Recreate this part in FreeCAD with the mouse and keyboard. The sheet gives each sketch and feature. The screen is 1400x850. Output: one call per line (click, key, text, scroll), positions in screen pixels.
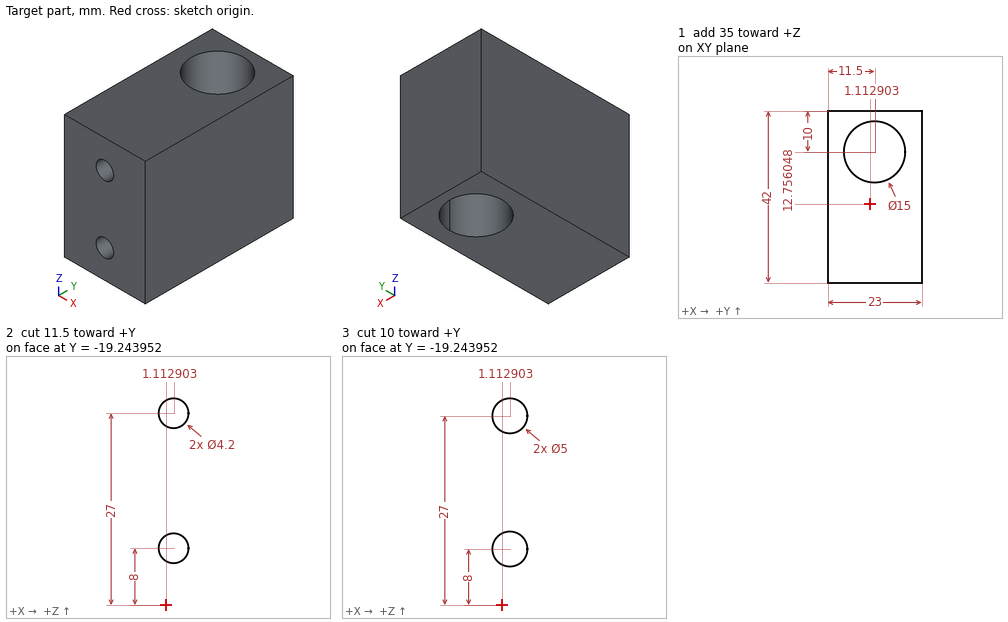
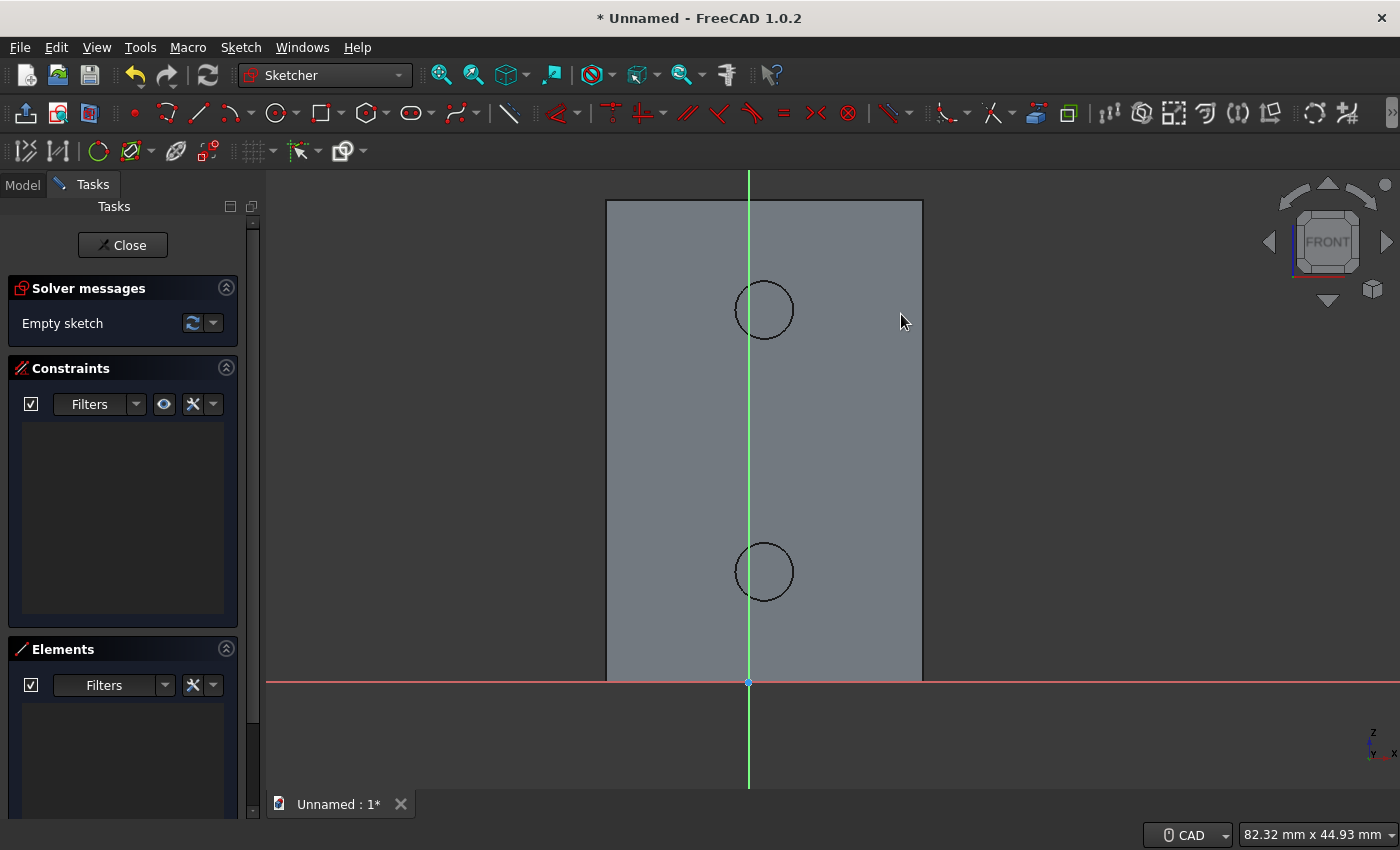
click(276, 114)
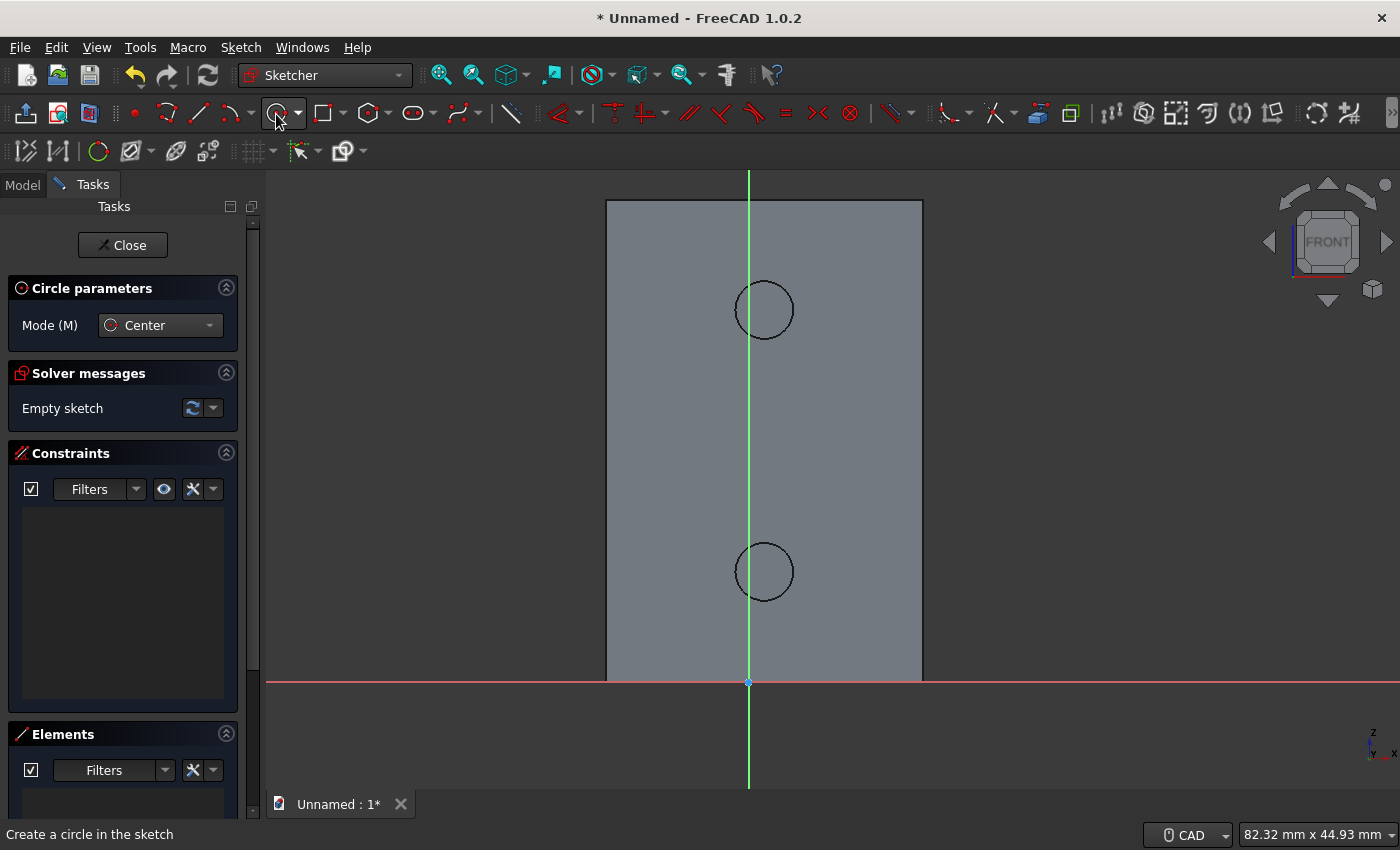
click(764, 310)
click(789, 286)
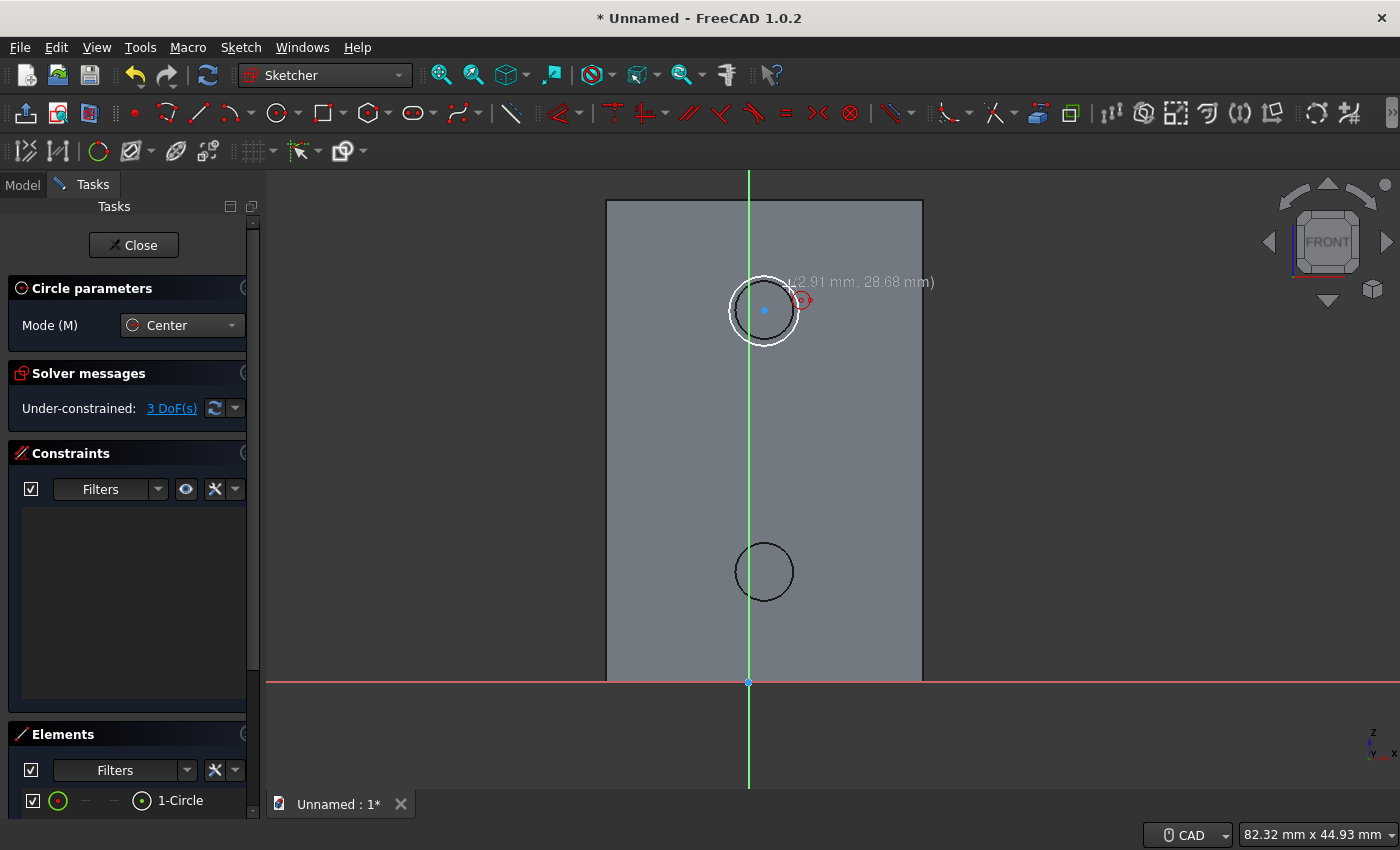
click(764, 572)
click(789, 547)
key(Escape)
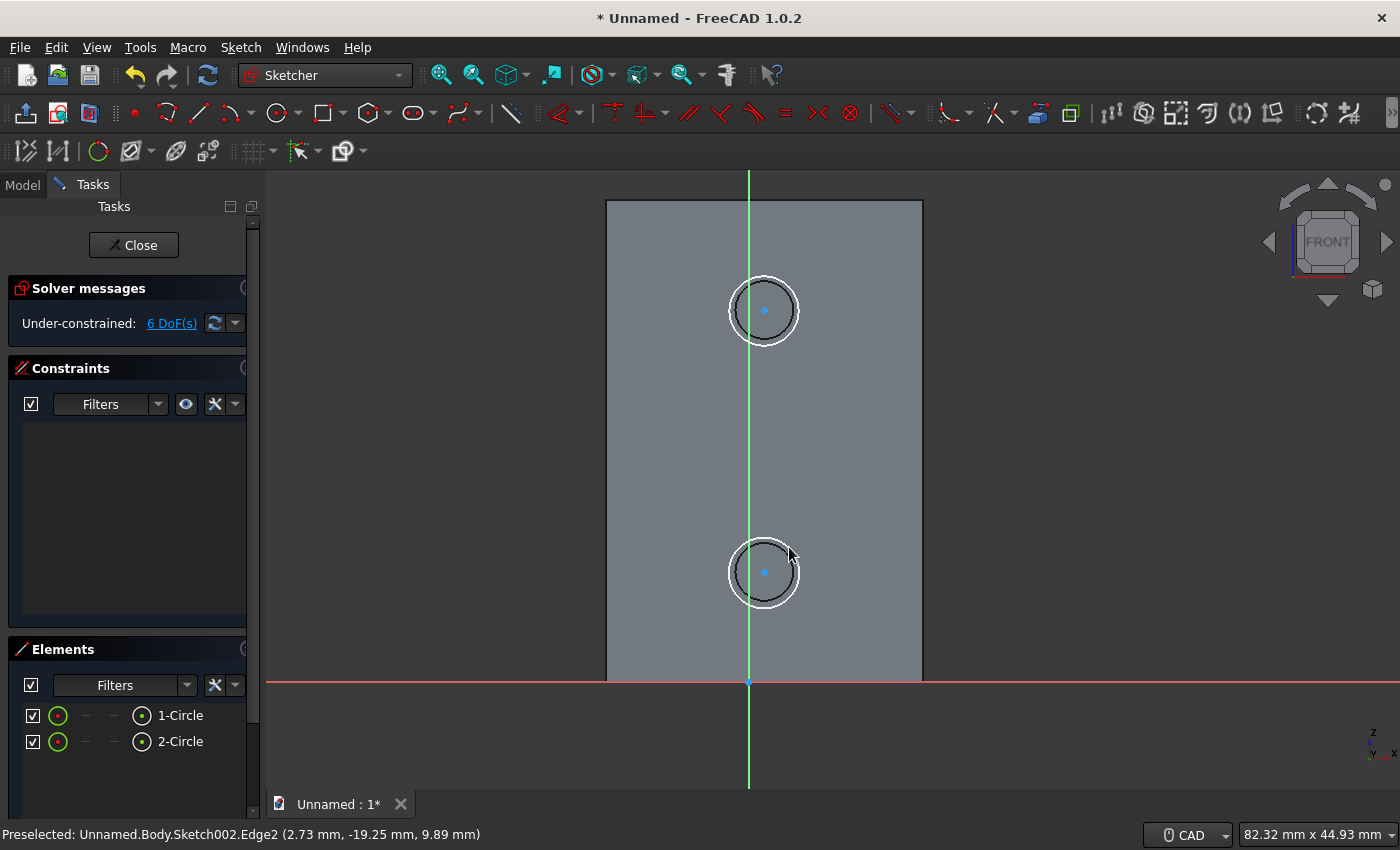
click(788, 286)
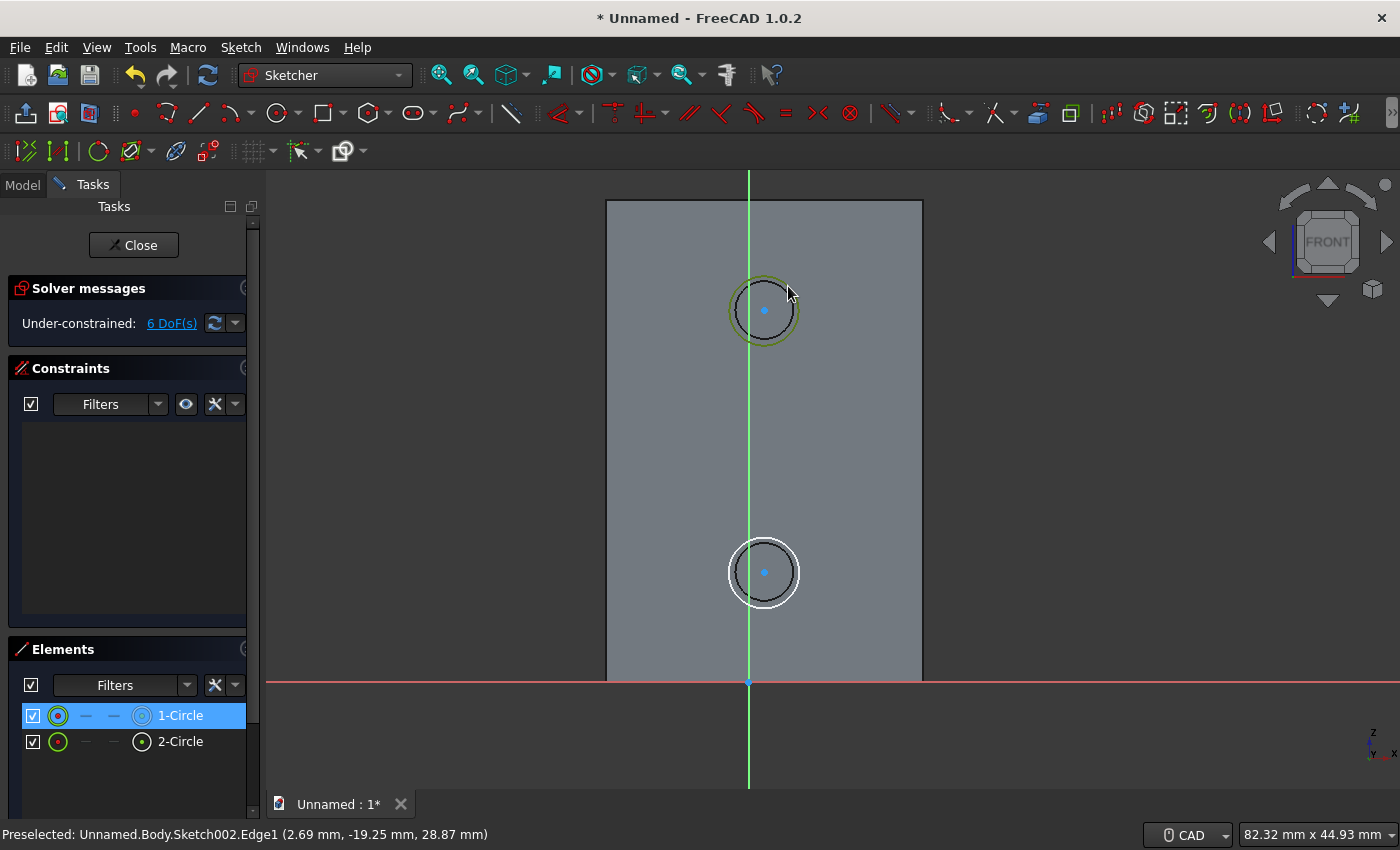
click(789, 548)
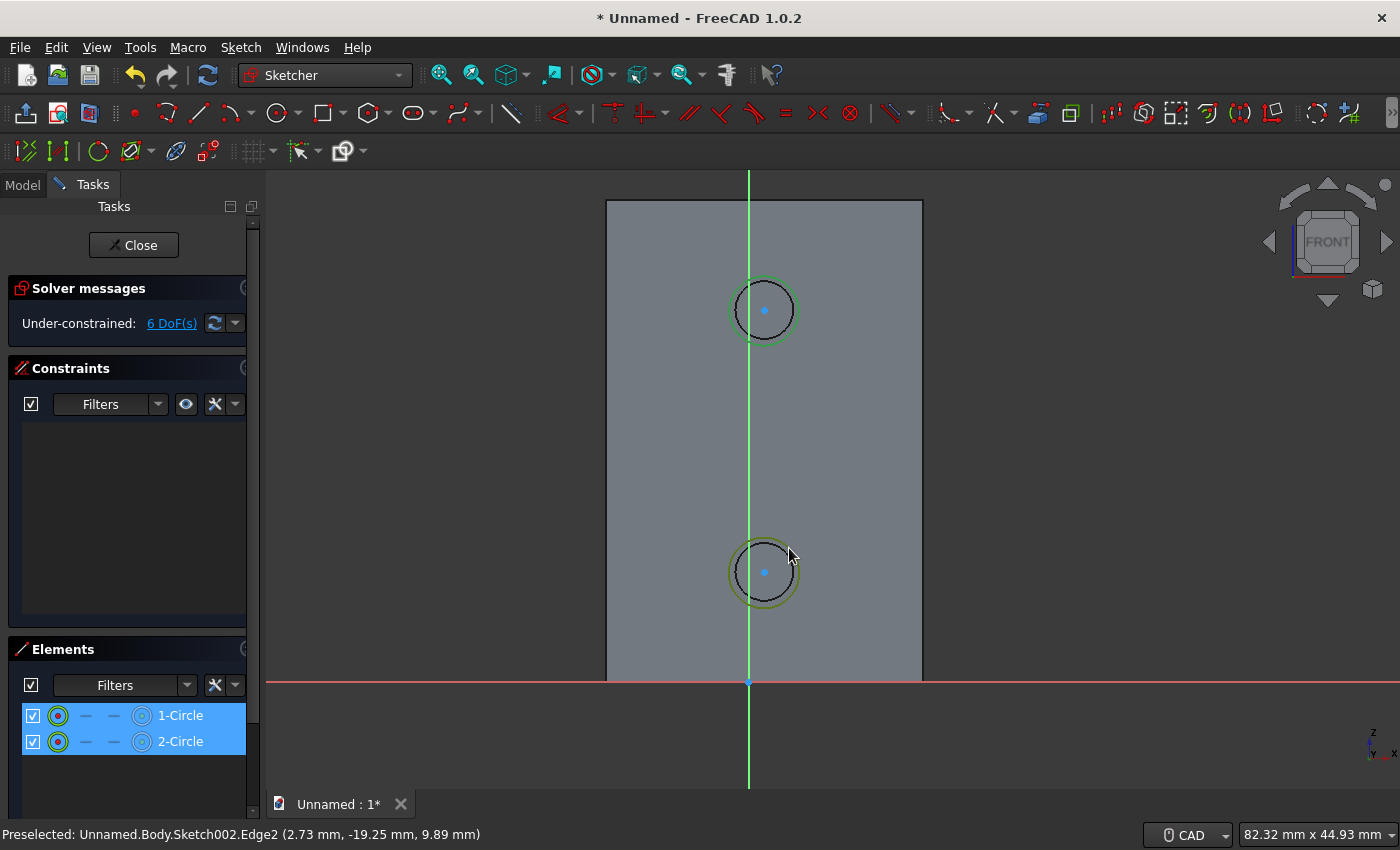
click(786, 114)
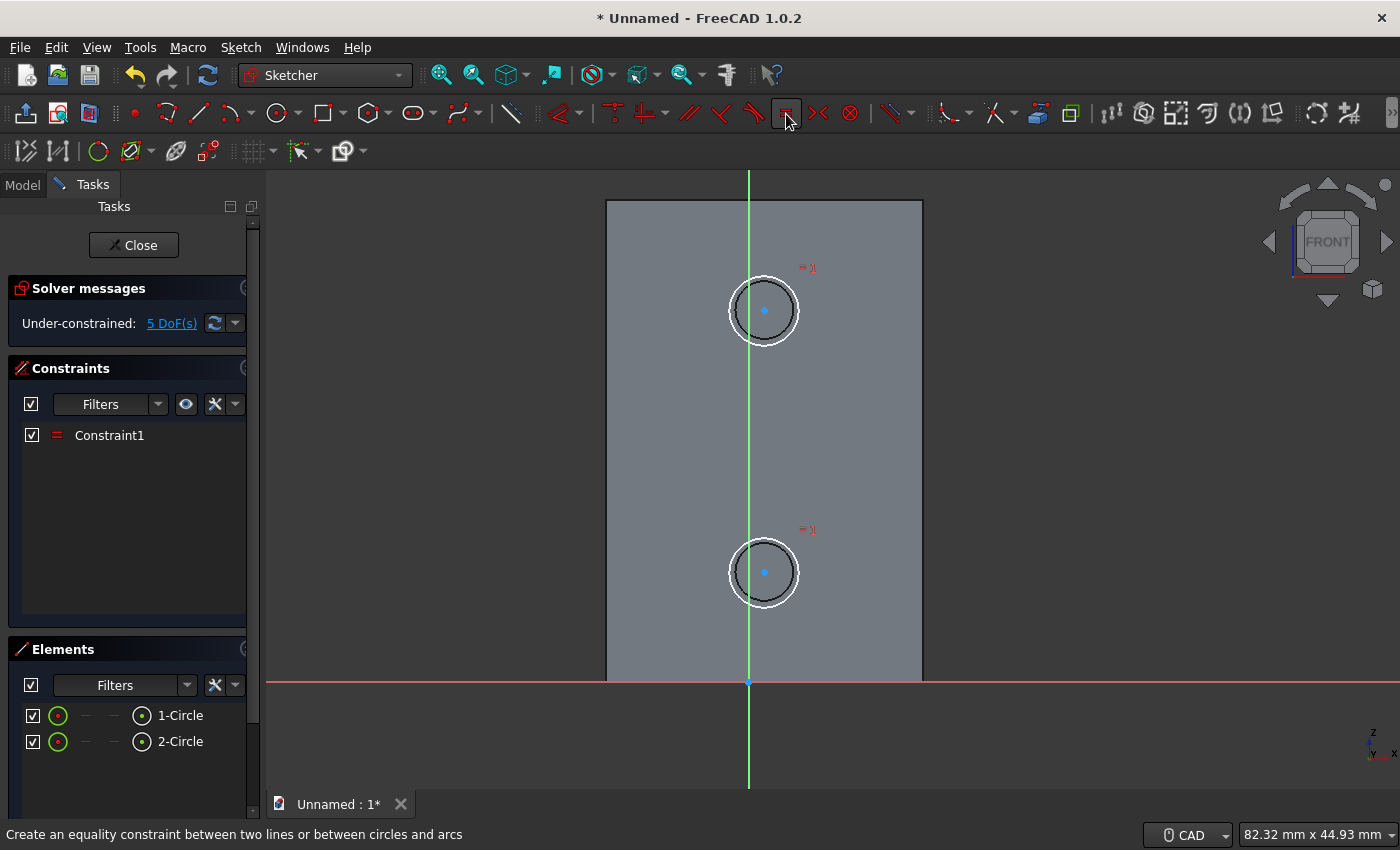
click(764, 311)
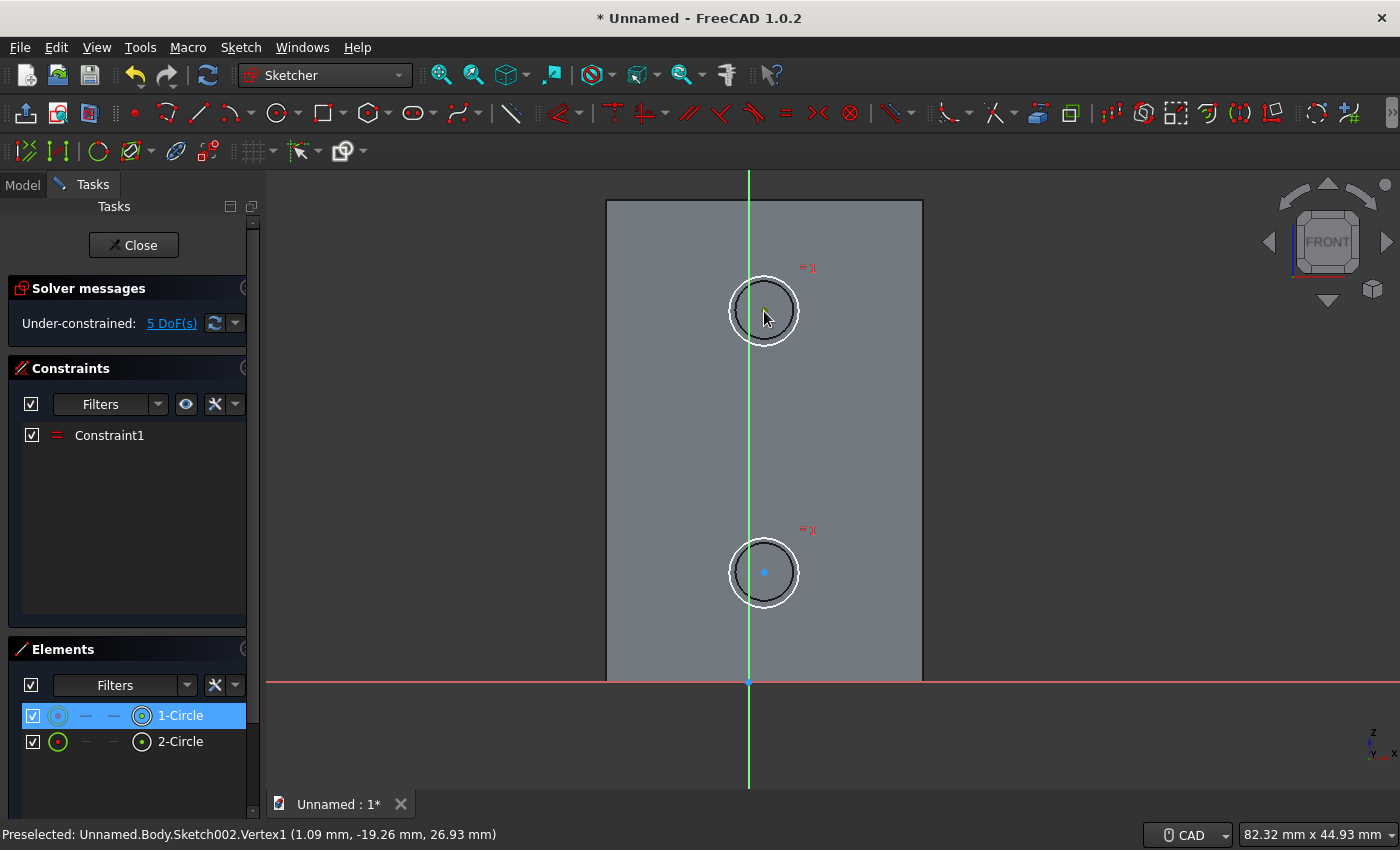
click(764, 573)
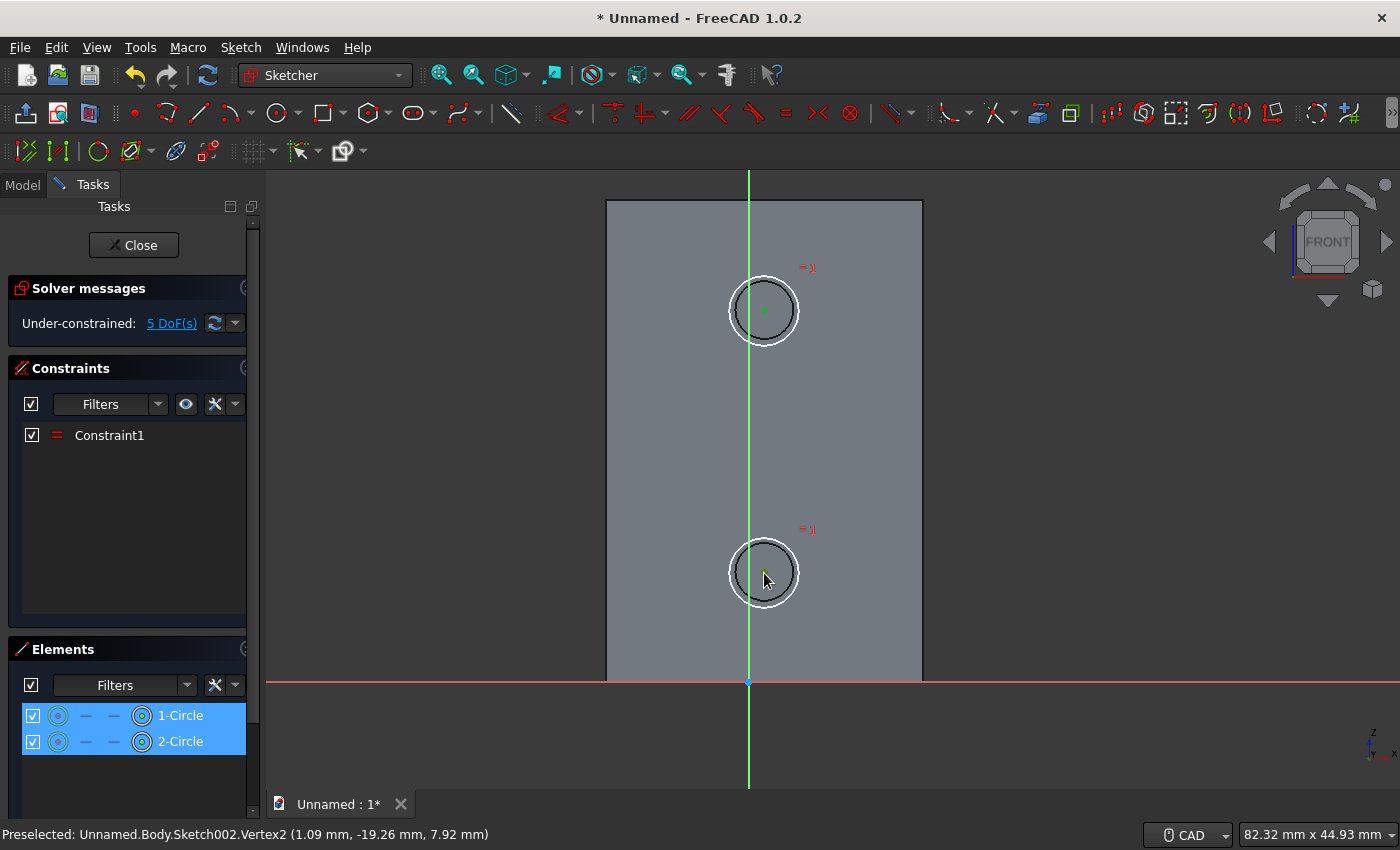
click(668, 114)